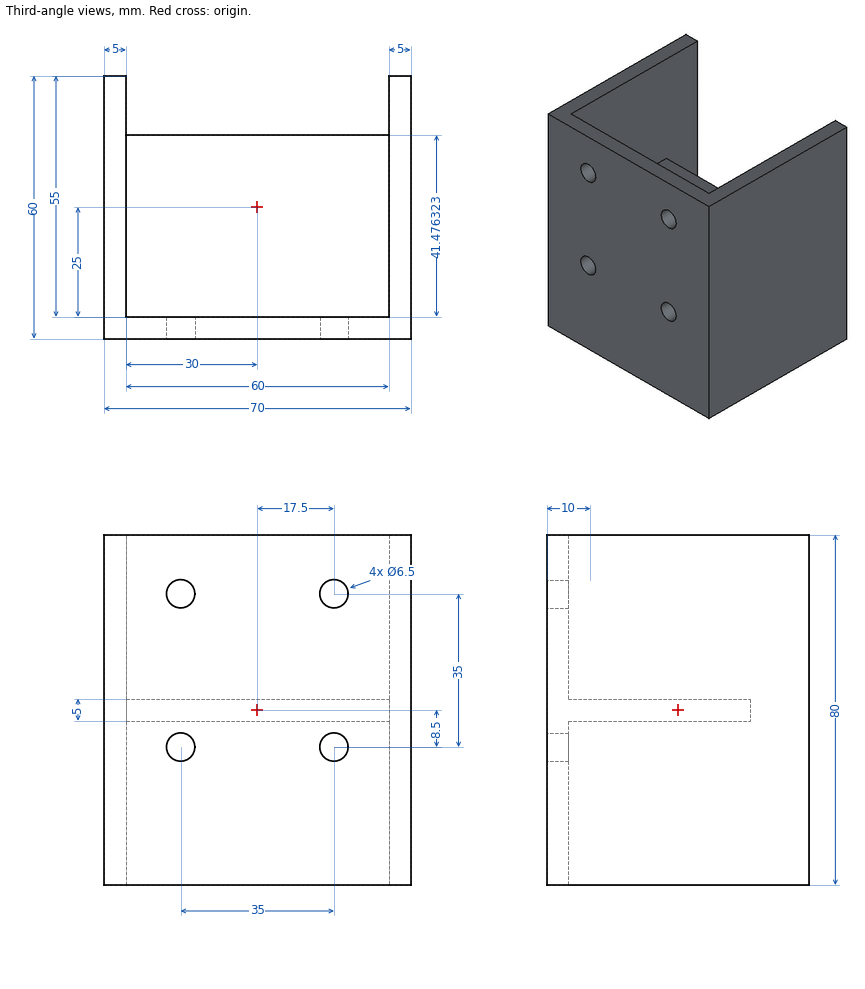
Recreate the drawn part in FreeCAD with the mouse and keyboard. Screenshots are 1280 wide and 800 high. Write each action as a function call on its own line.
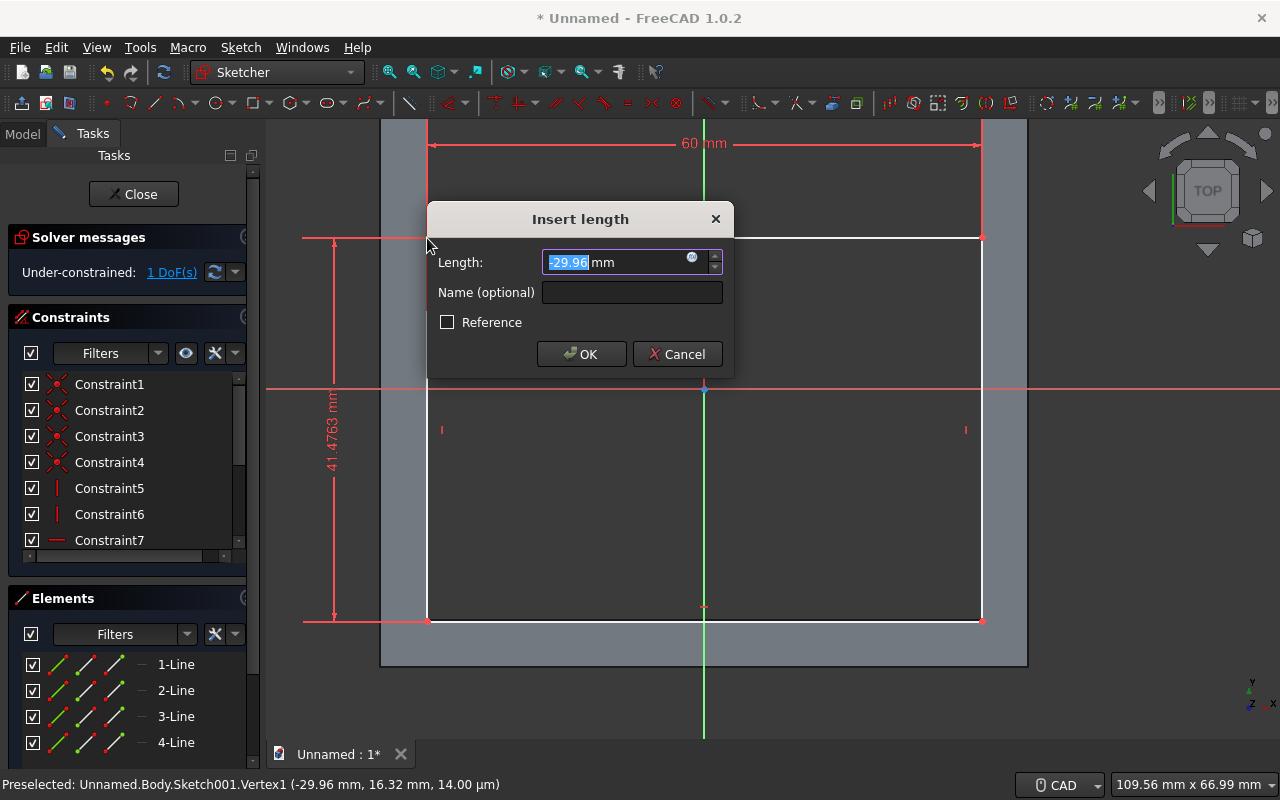
text(-30)
key(Return)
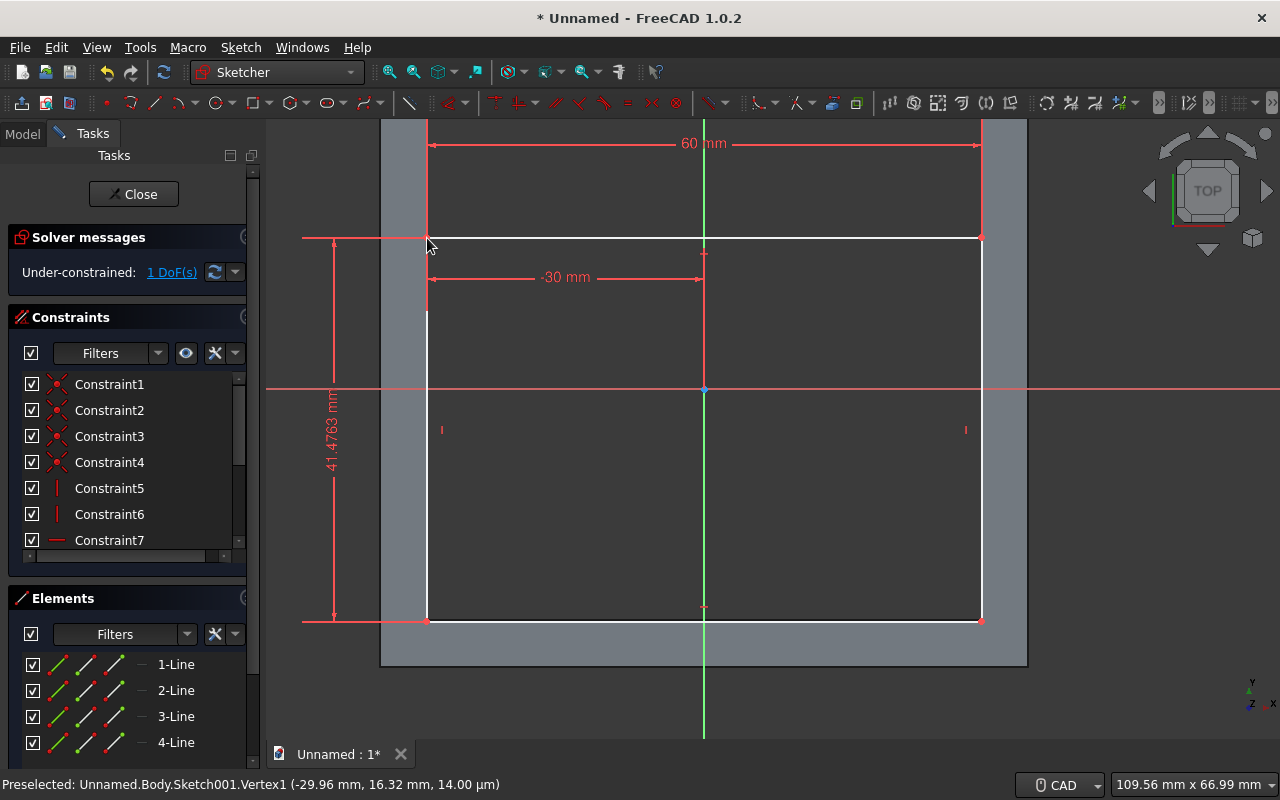
click(427, 622)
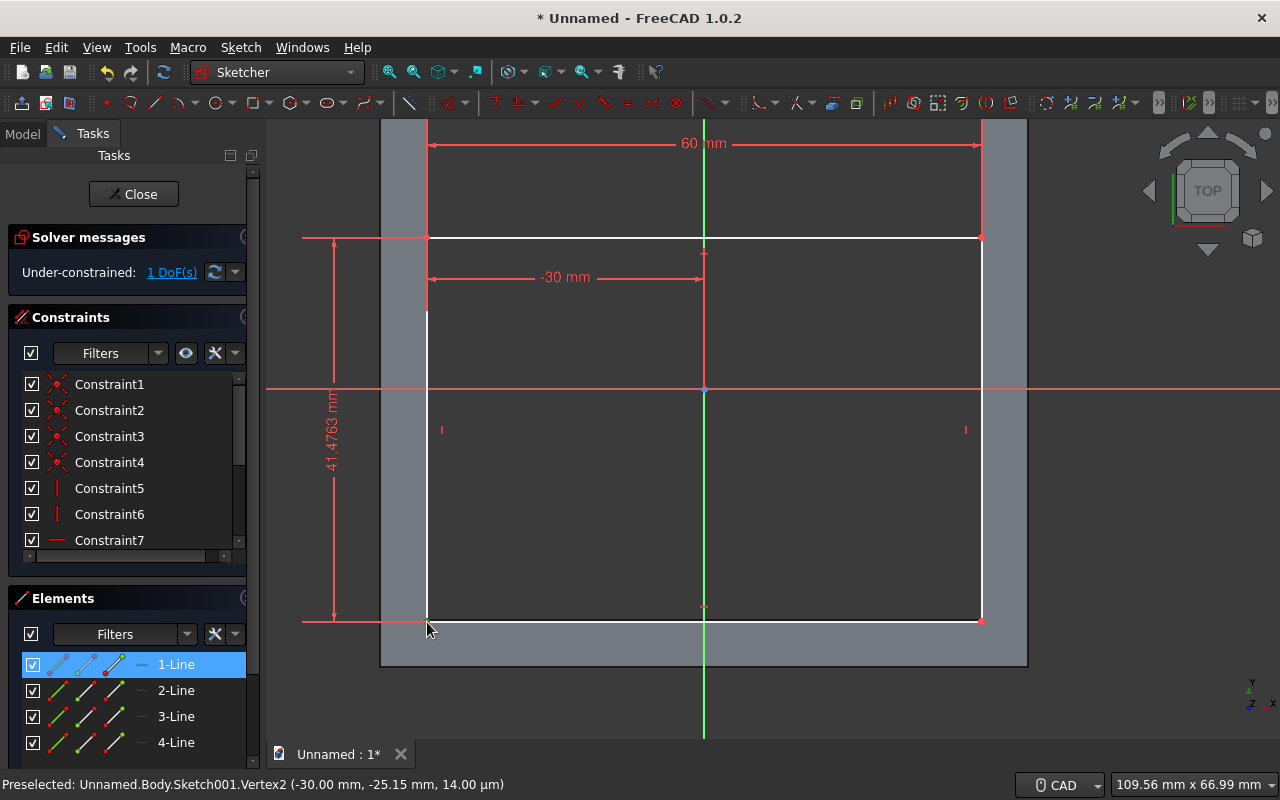
key(i)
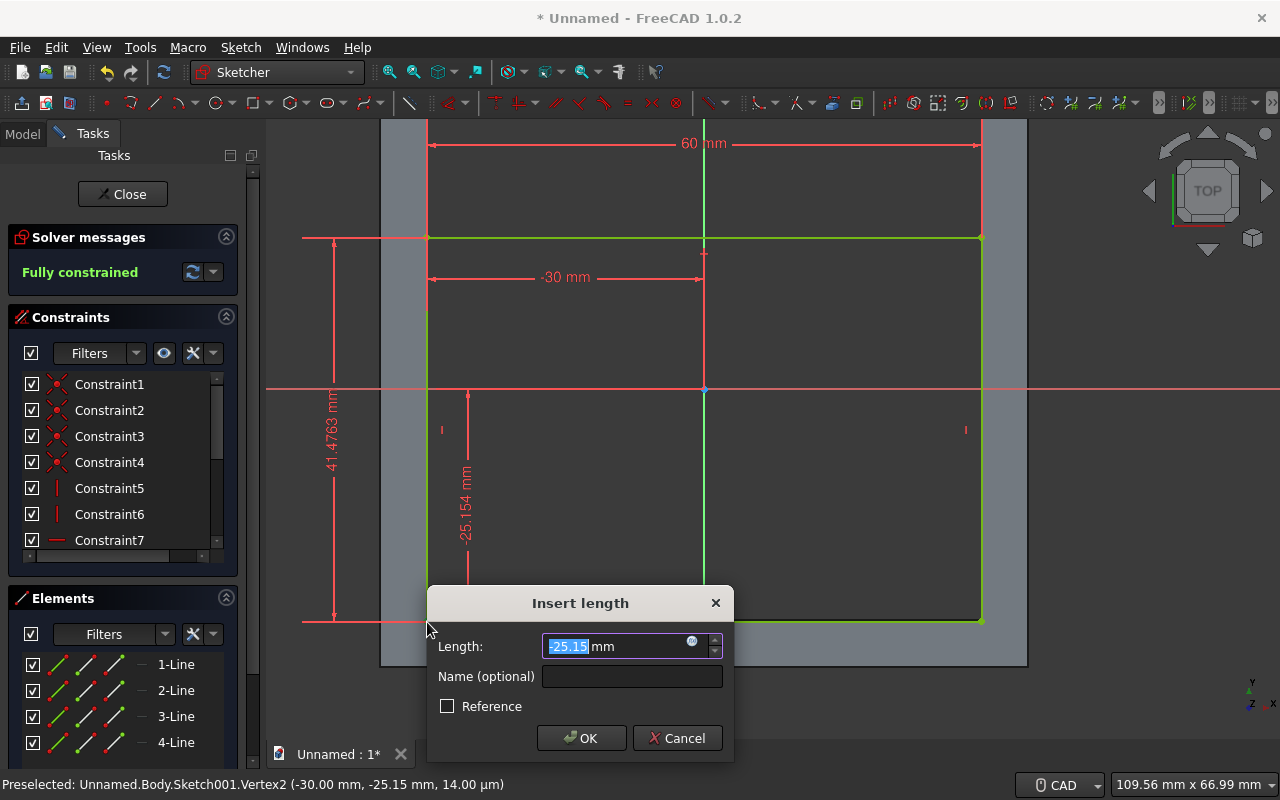
text(-25)
key(Return)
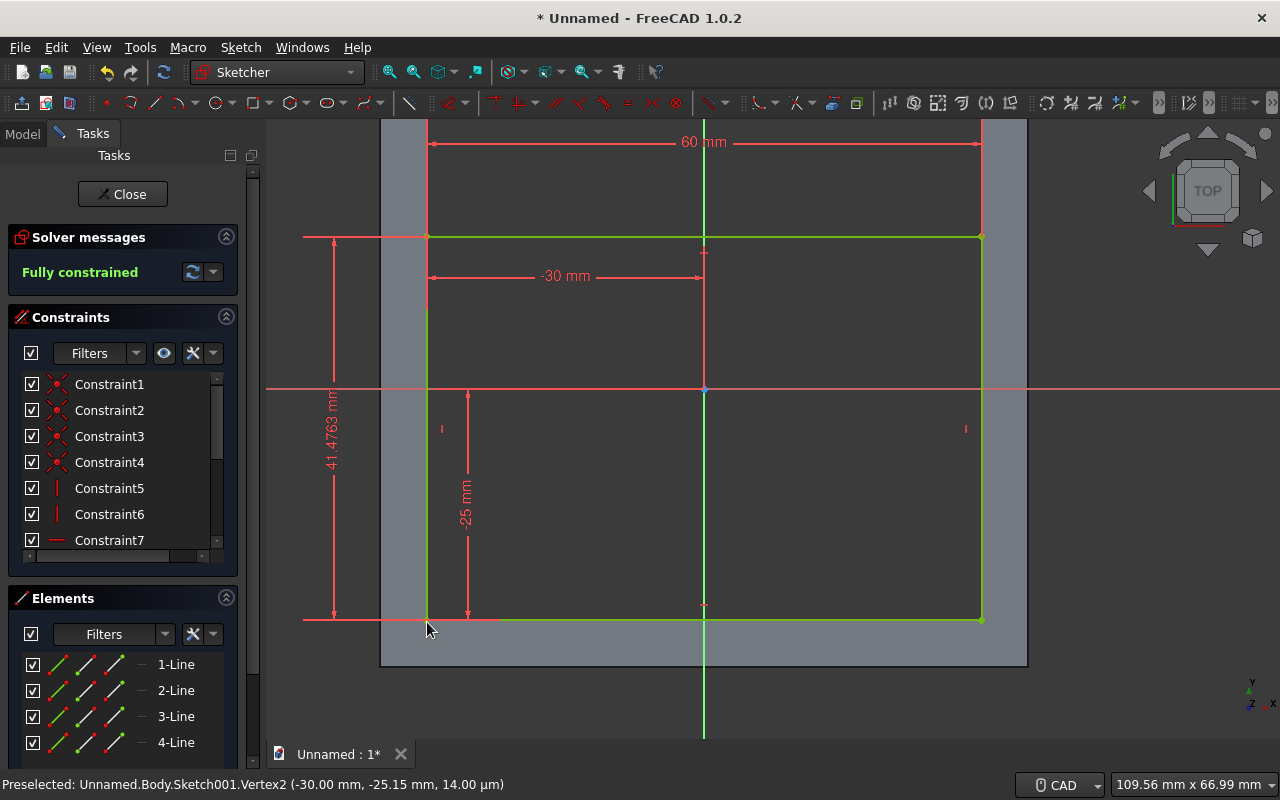
click(123, 194)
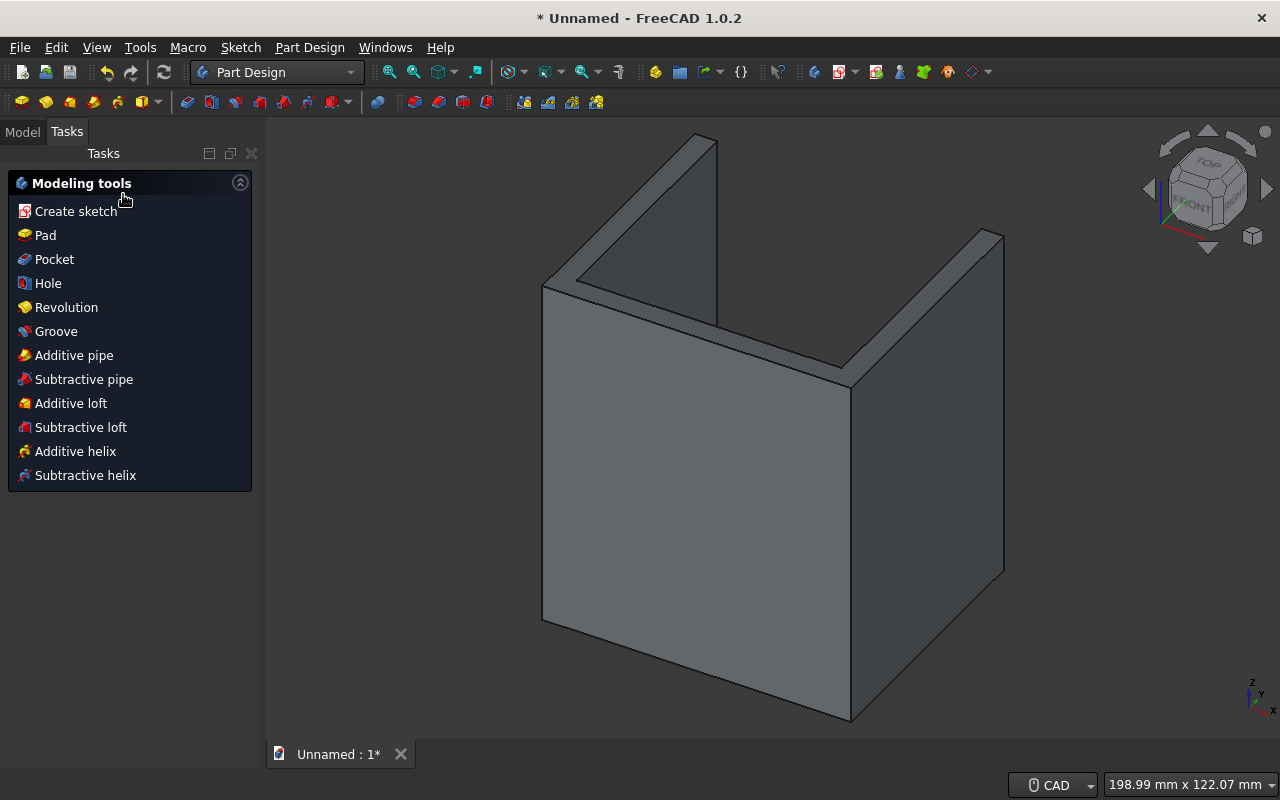
click(22, 102)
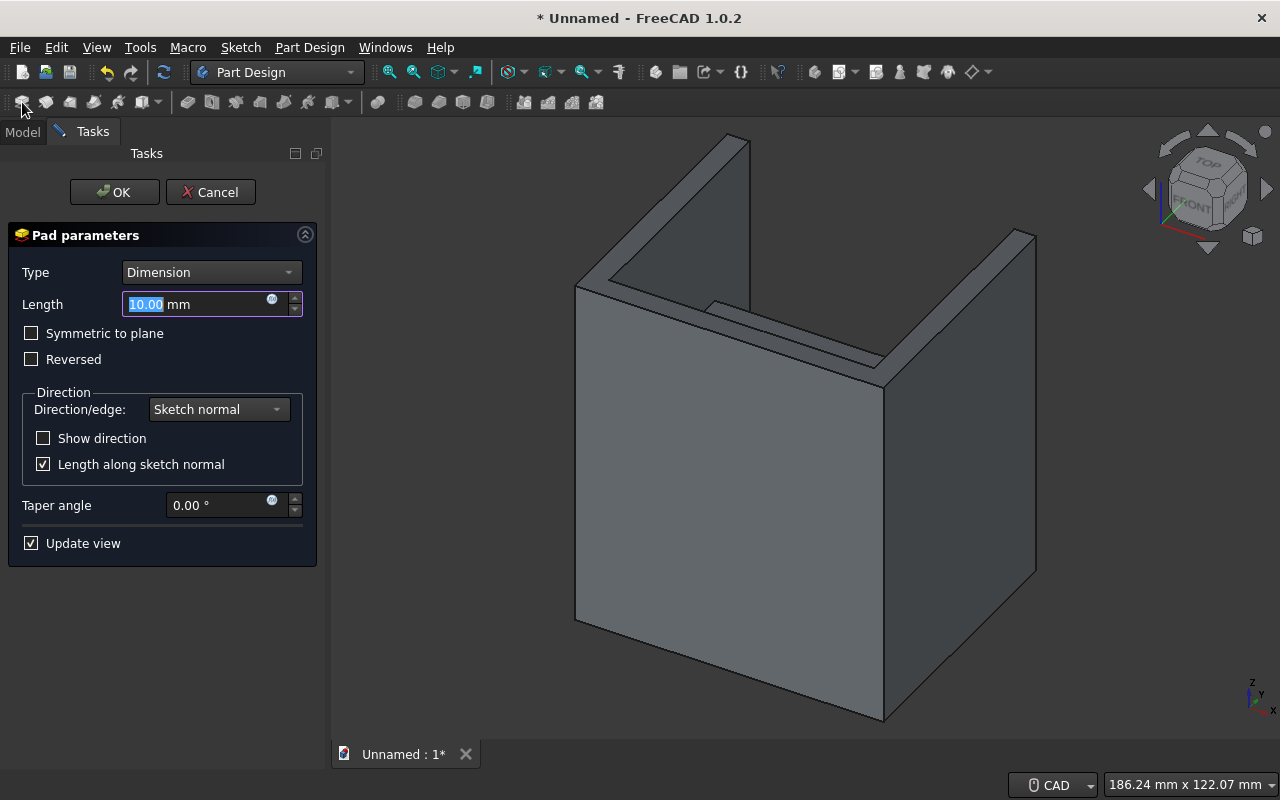
text(5)
key(Tab)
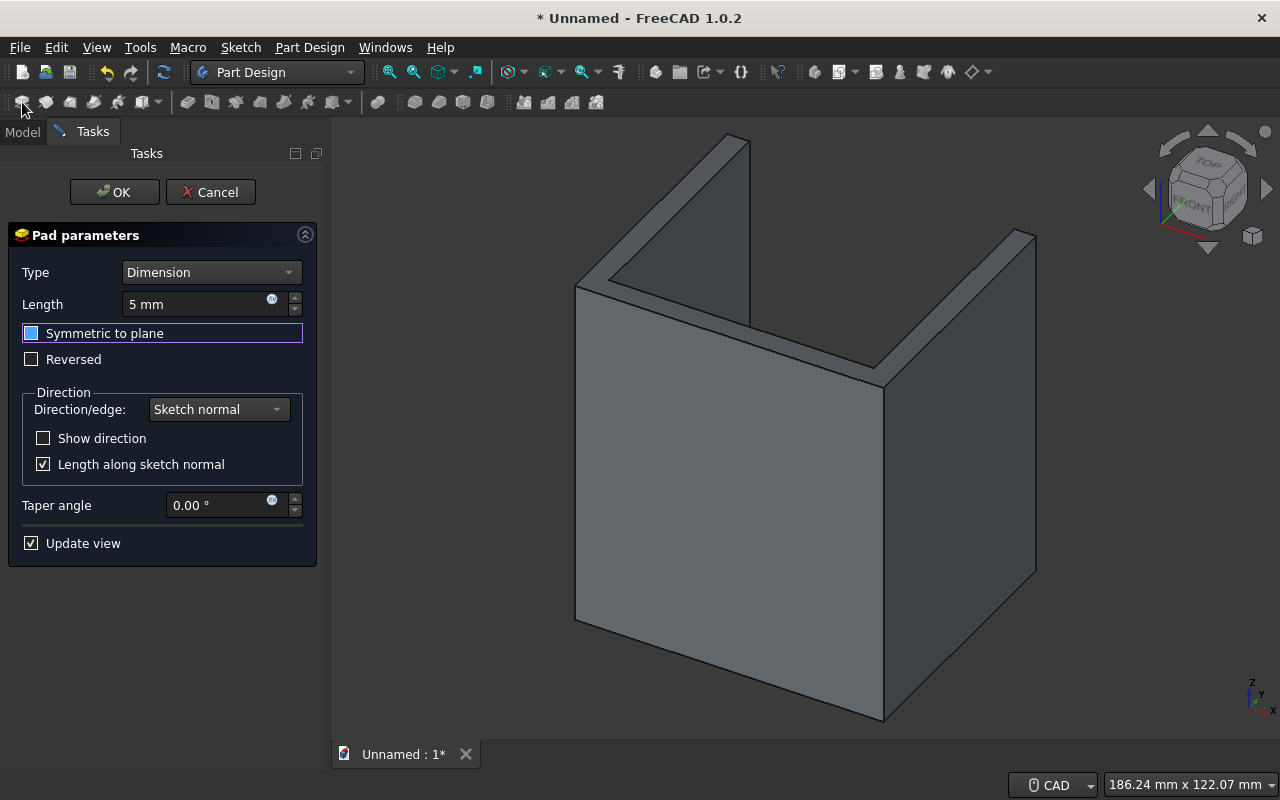
click(30, 333)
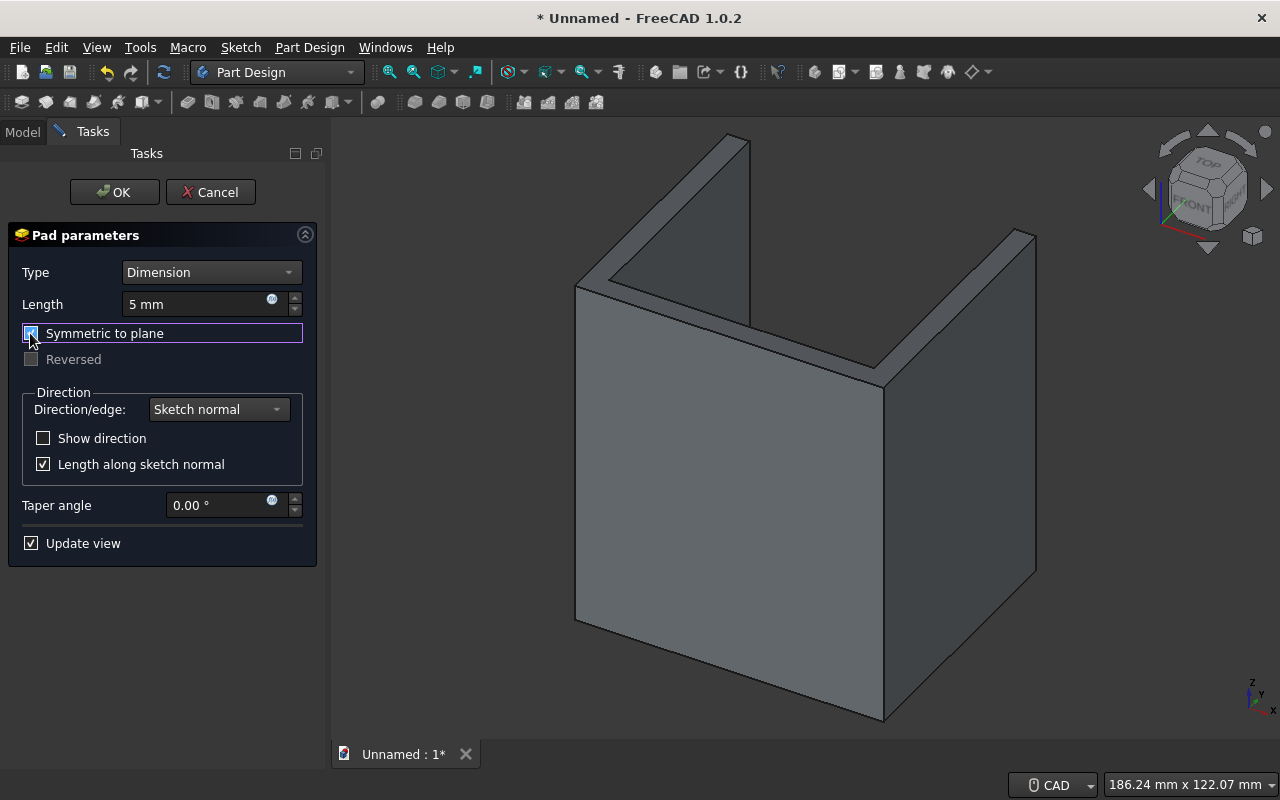
click(115, 192)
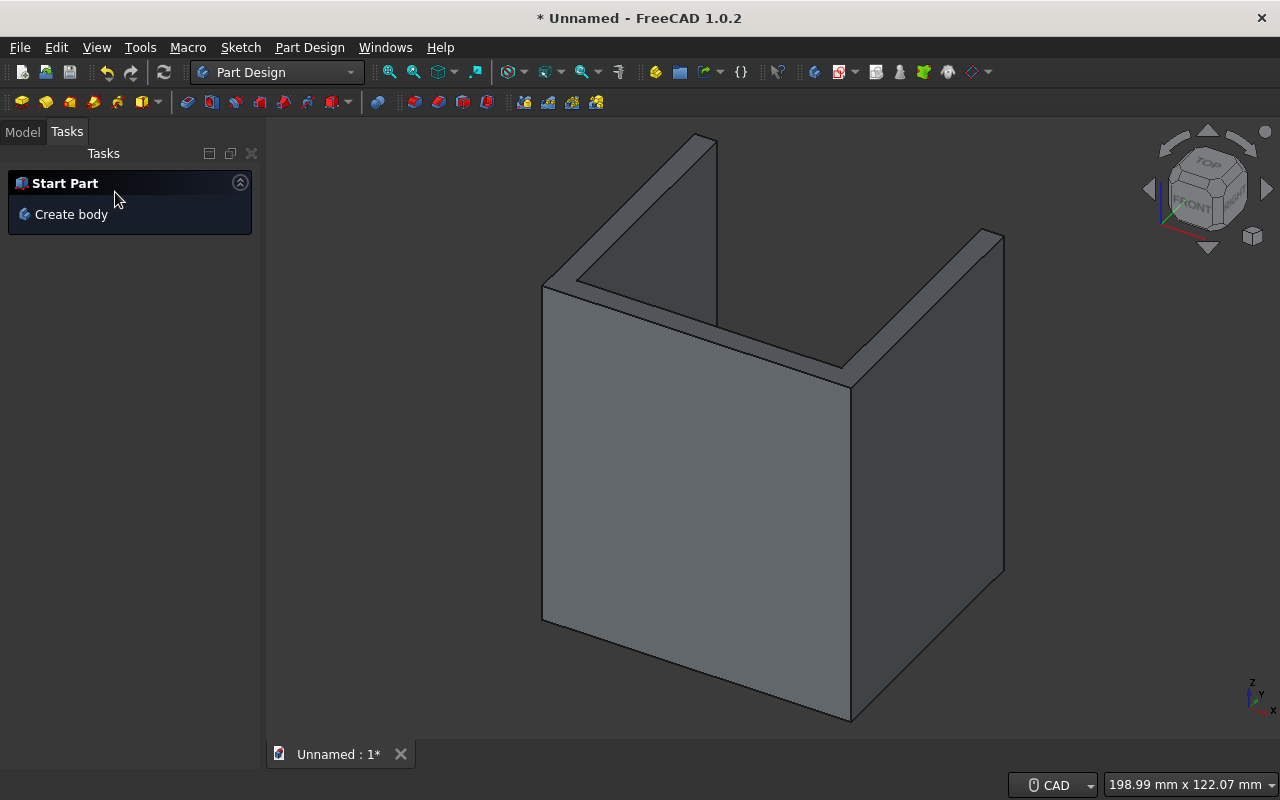
click(697, 503)